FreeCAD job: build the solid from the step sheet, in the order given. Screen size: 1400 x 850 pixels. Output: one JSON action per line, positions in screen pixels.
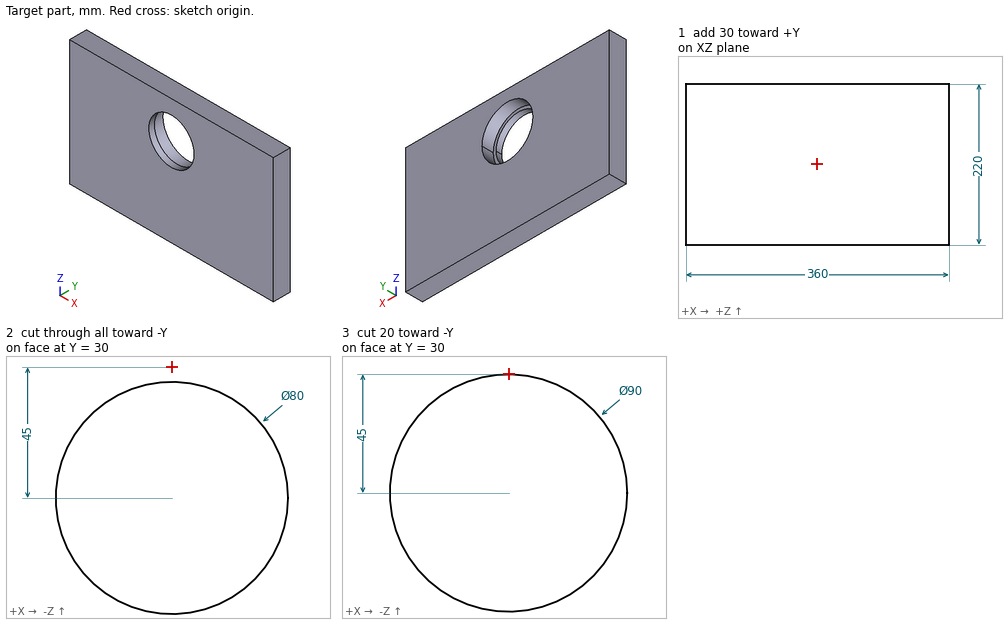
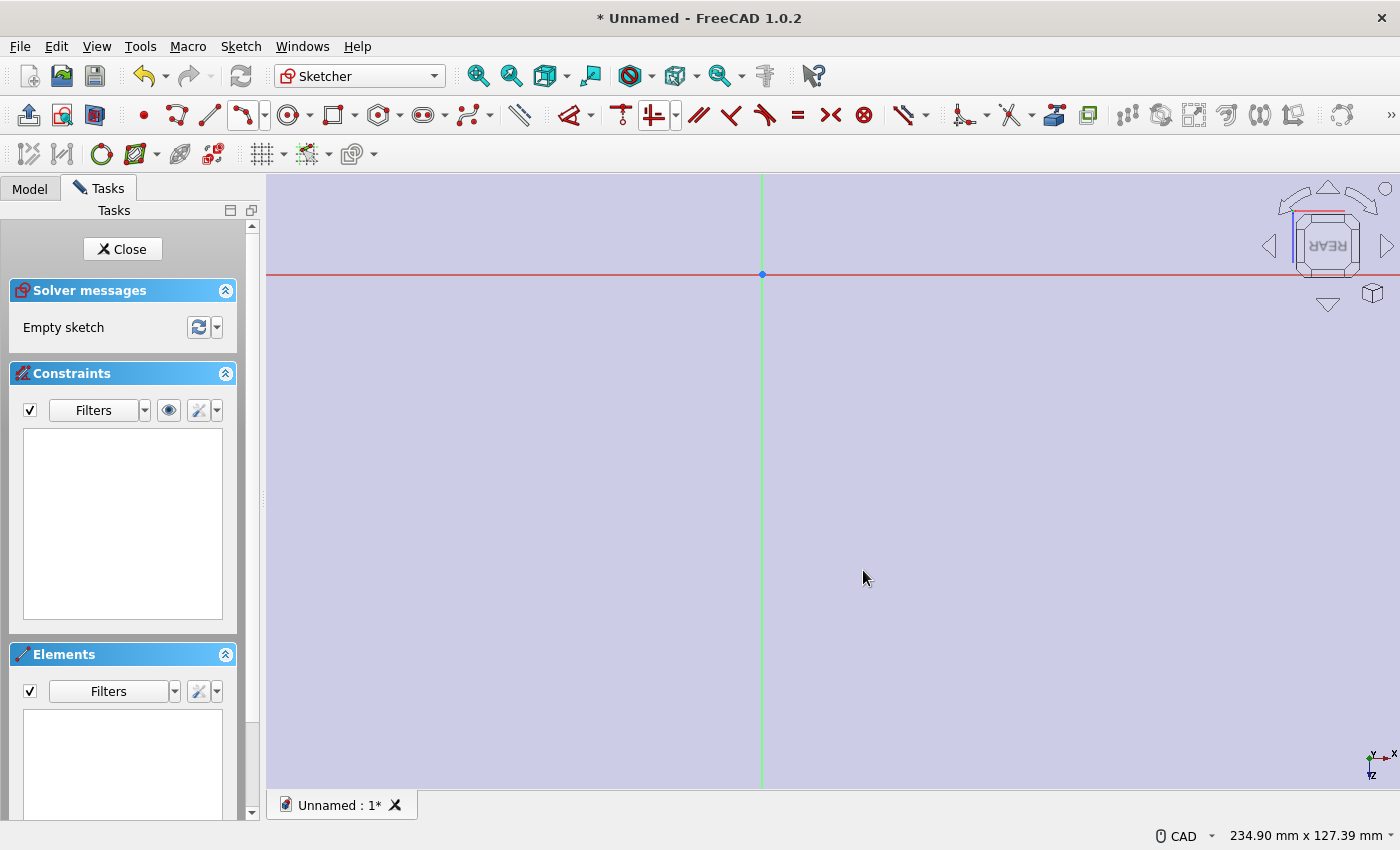
{"action": "left_click", "coordinate": [288, 116]}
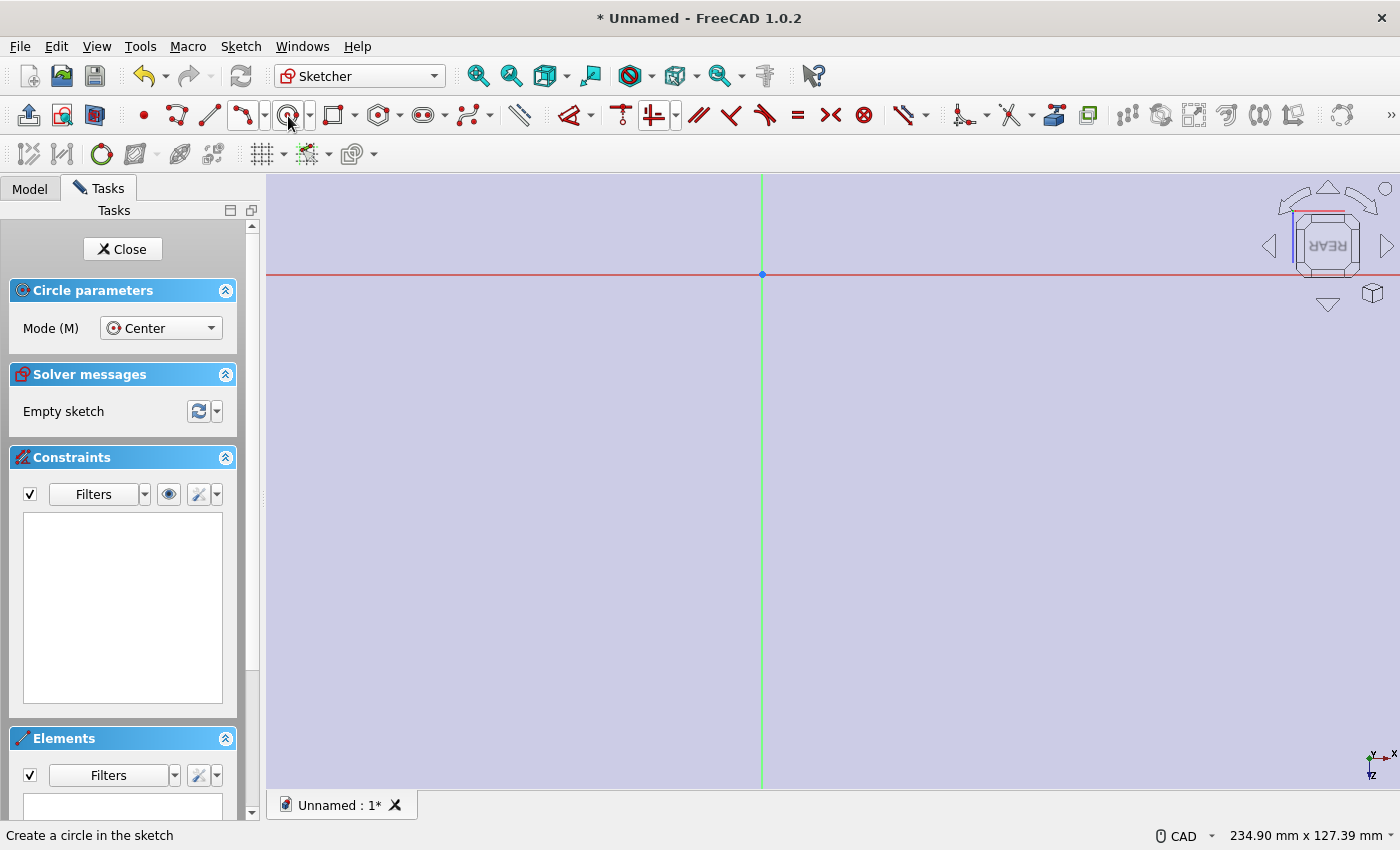
{"action": "left_click", "coordinate": [762, 492]}
{"action": "mouse_move", "coordinate": [899, 355]}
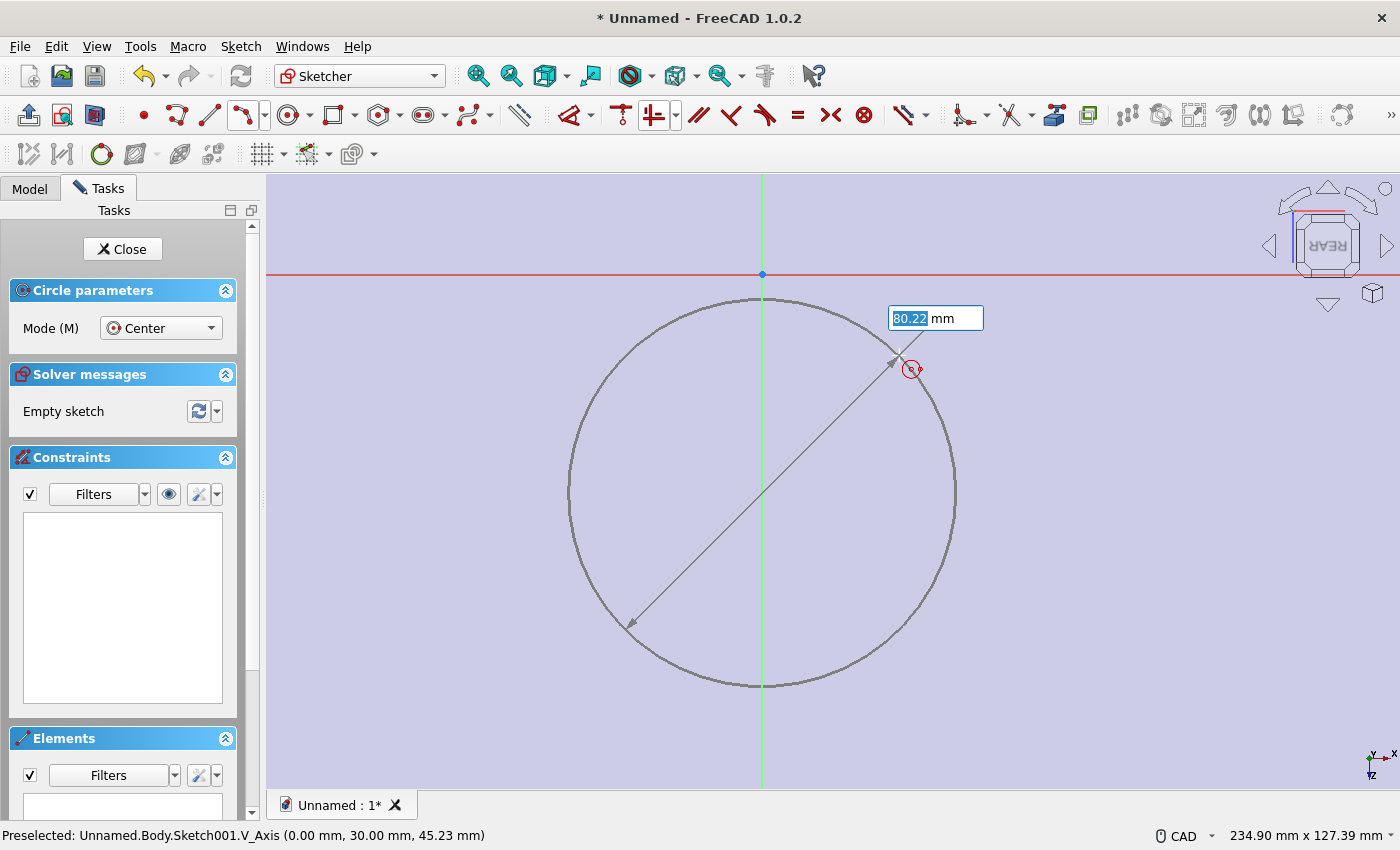
{"action": "type", "text": "80"}
{"action": "key", "text": "Return"}
{"action": "key", "text": "Escape"}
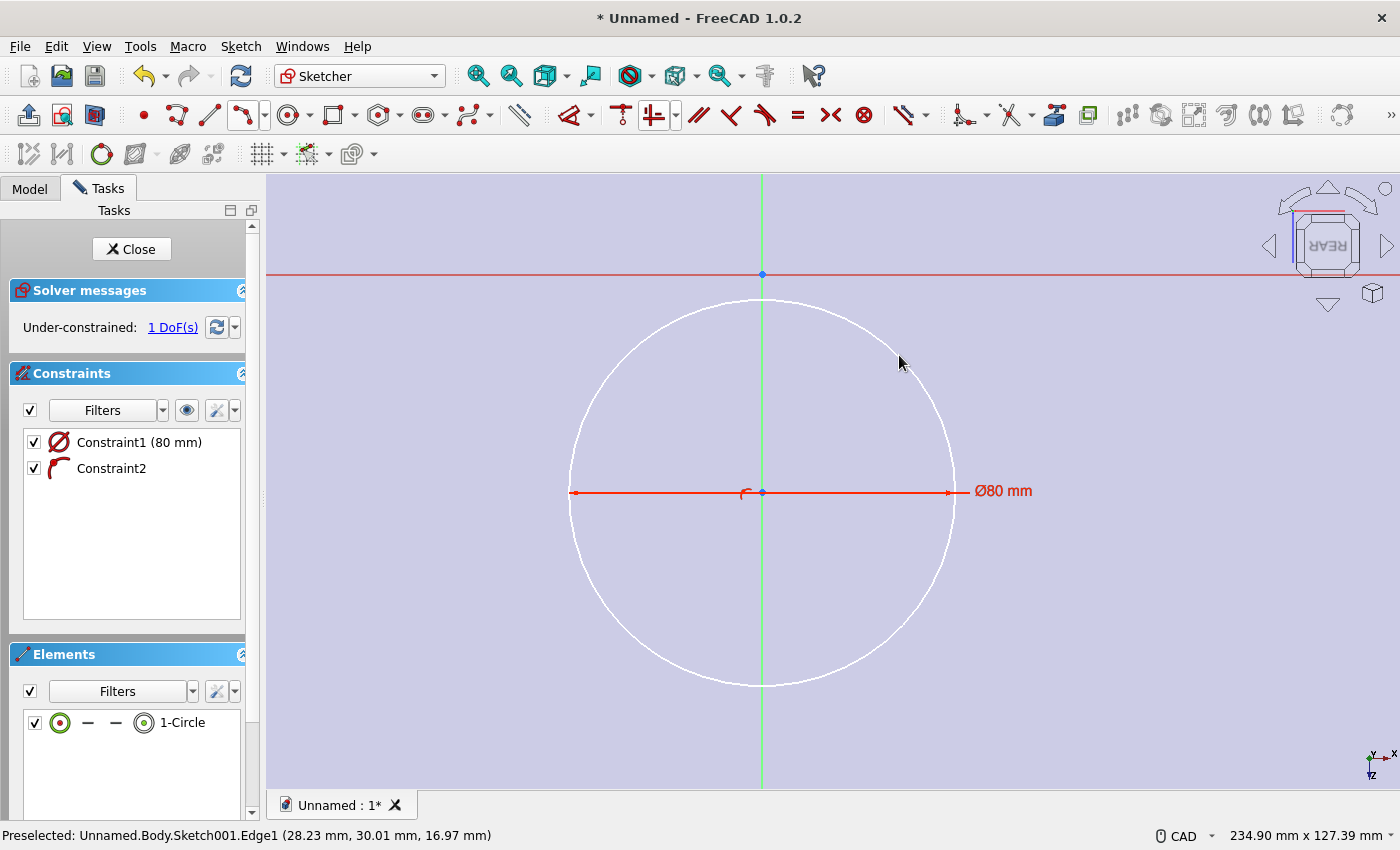
{"action": "left_click", "coordinate": [568, 116]}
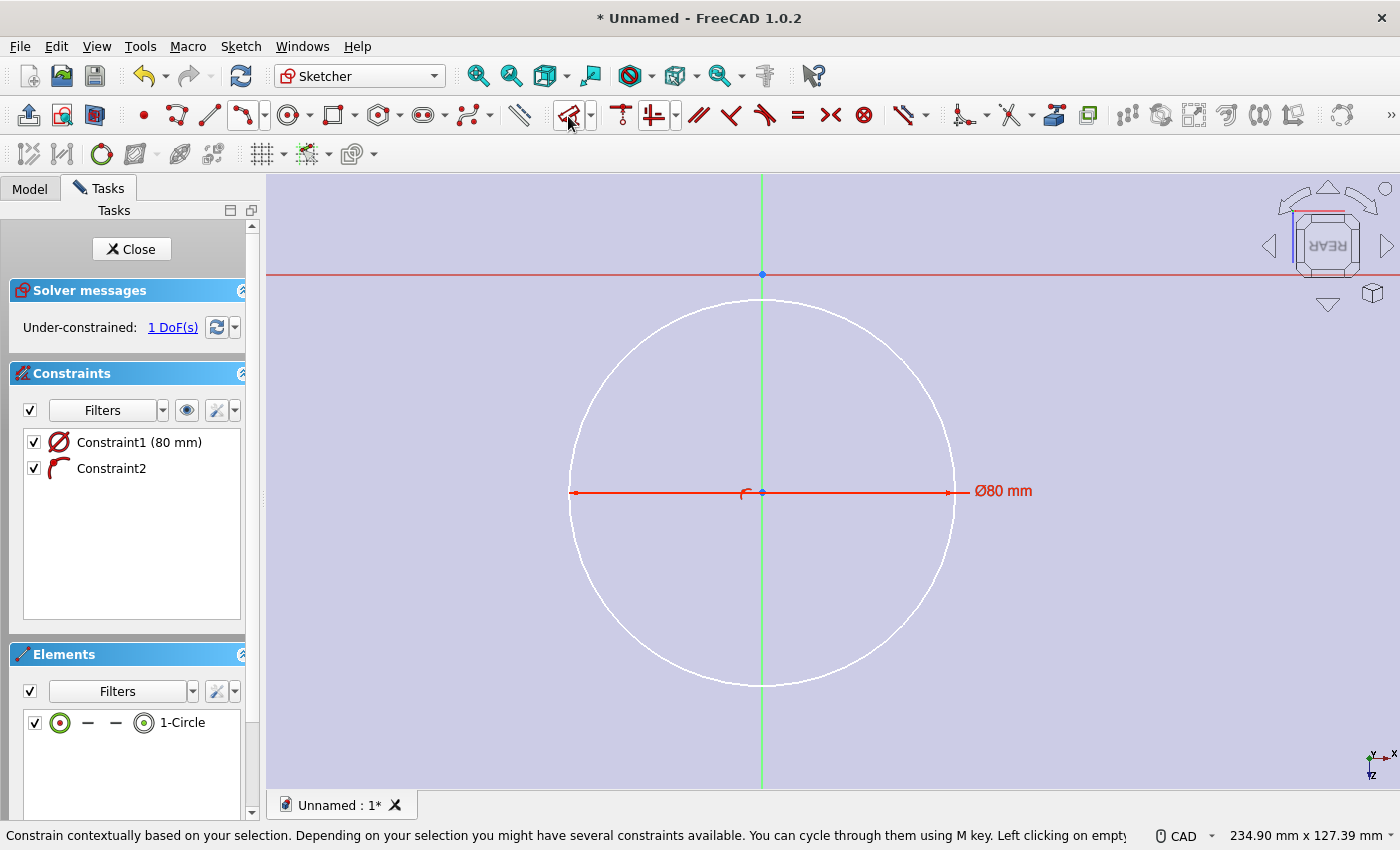
{"action": "left_click", "coordinate": [762, 493]}
{"action": "left_click", "coordinate": [796, 384]}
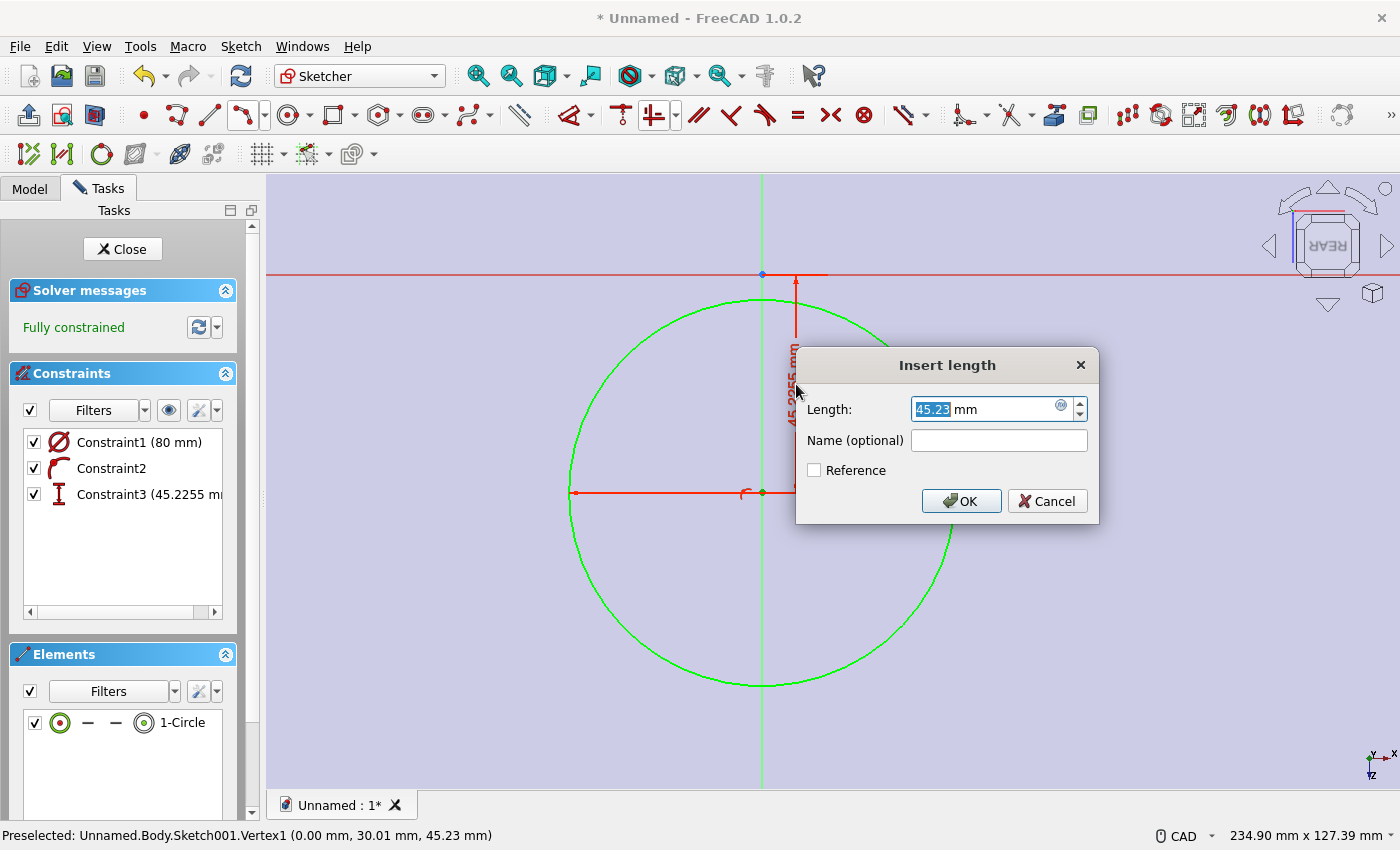
{"action": "type", "text": "45"}
{"action": "key", "text": "Return"}
{"action": "key", "text": "Escape"}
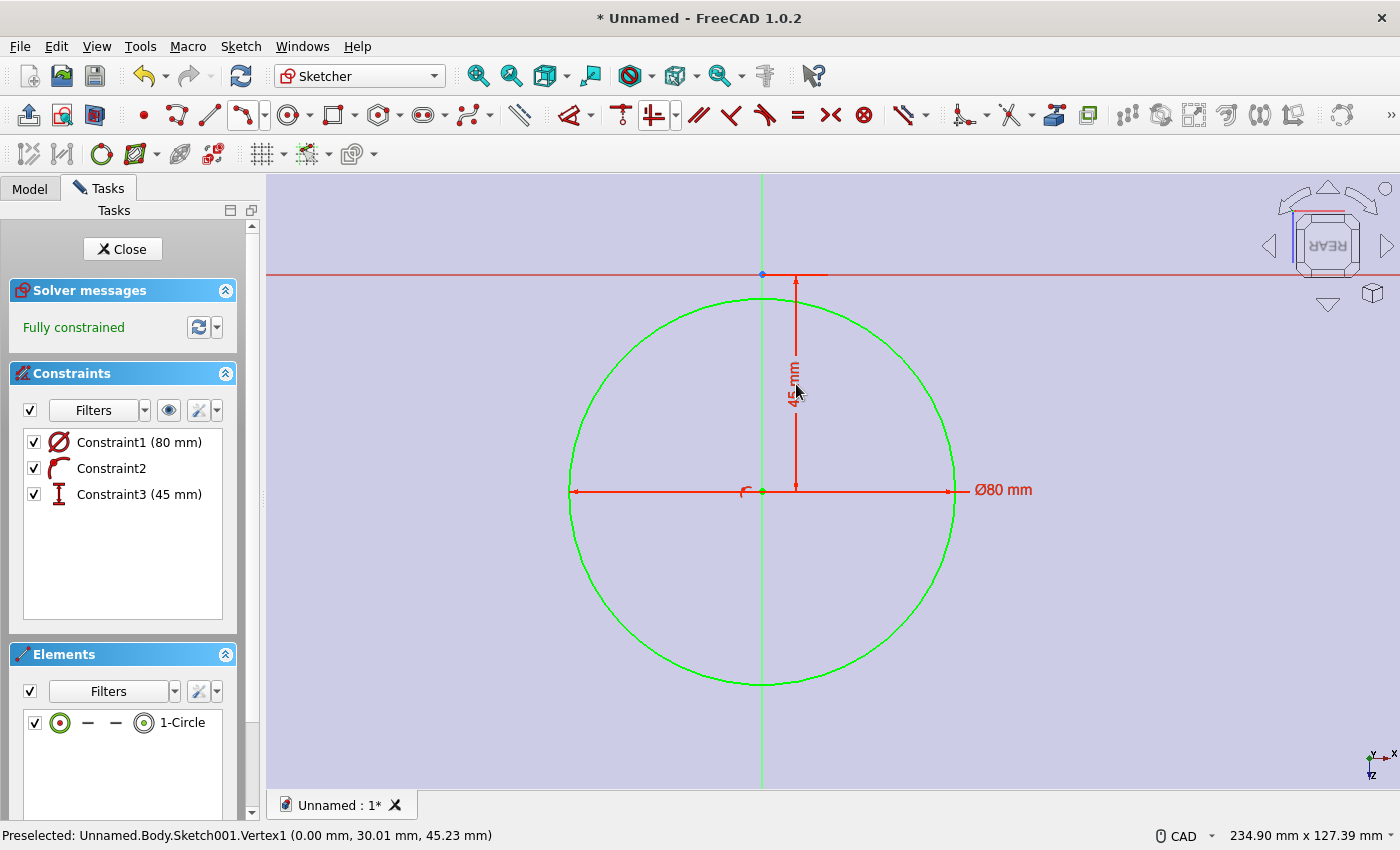
{"action": "left_click", "coordinate": [123, 249]}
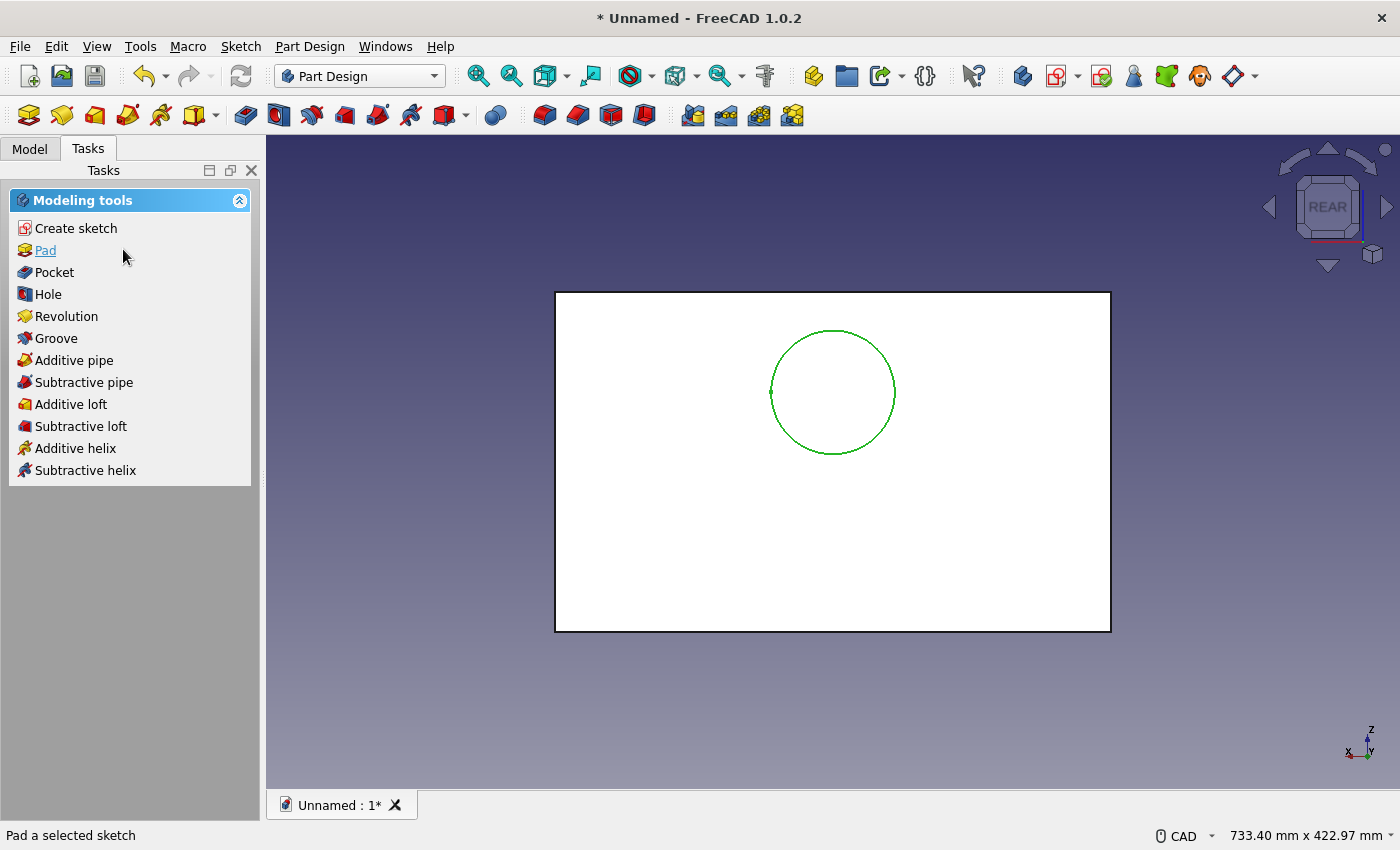
{"action": "left_click", "coordinate": [246, 116]}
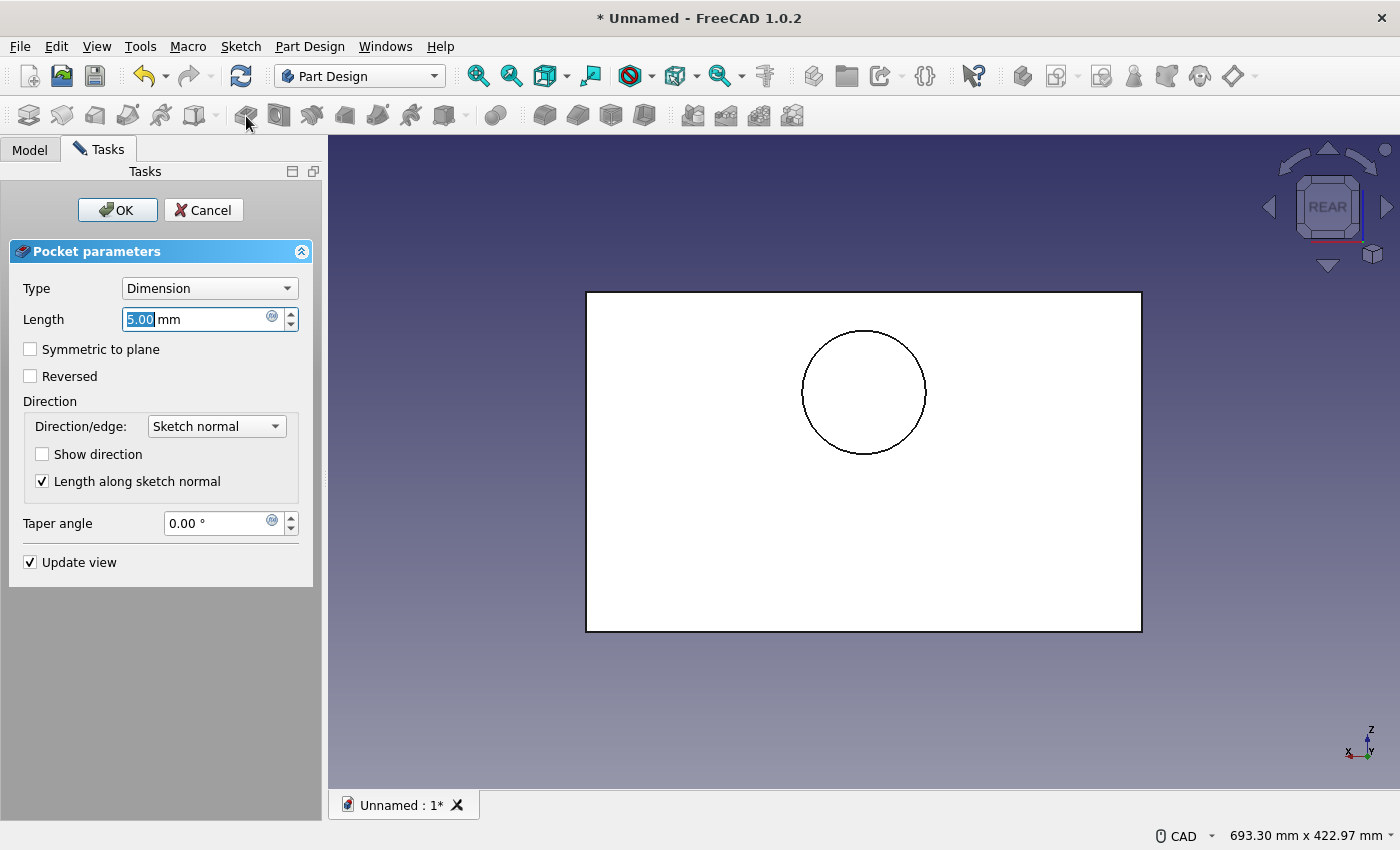
{"action": "left_click", "coordinate": [210, 288]}